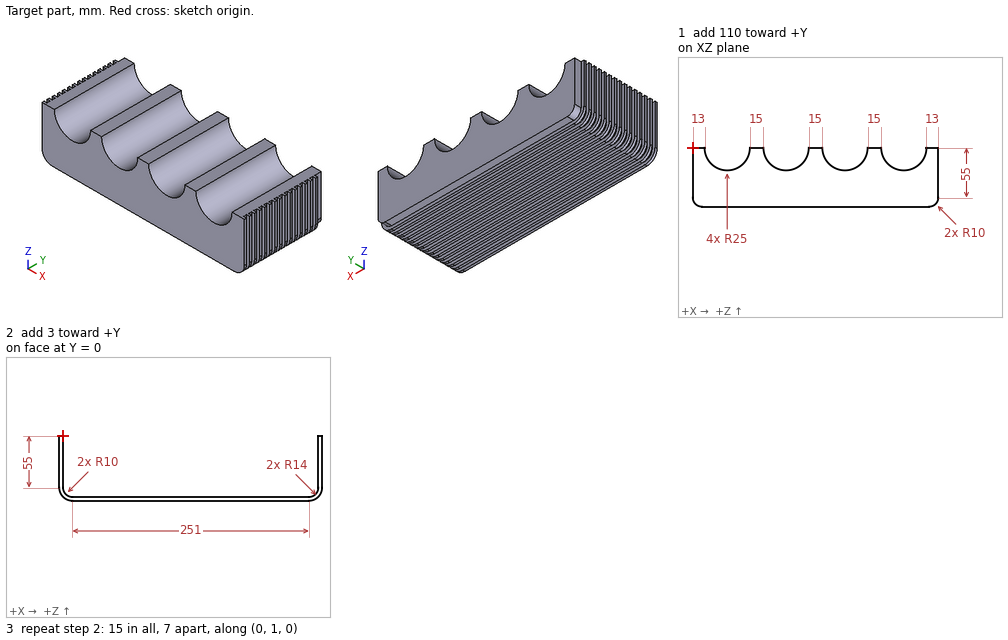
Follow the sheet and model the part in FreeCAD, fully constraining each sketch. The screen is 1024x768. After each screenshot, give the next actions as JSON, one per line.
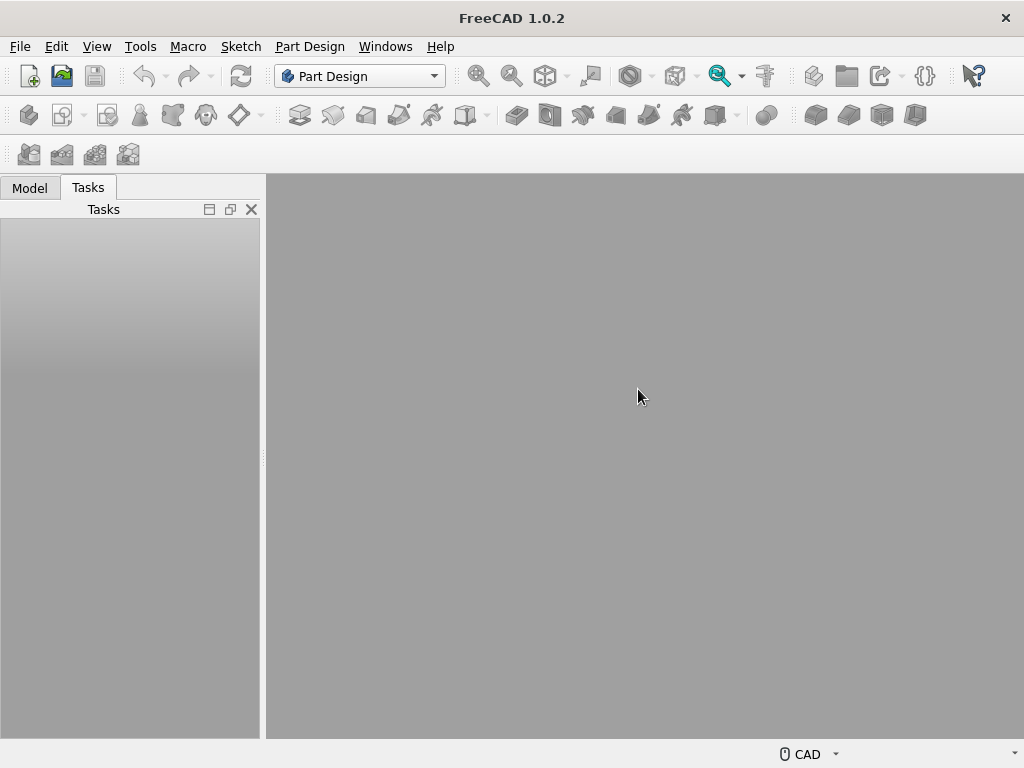
{"action": "left_click", "coordinate": [29, 76]}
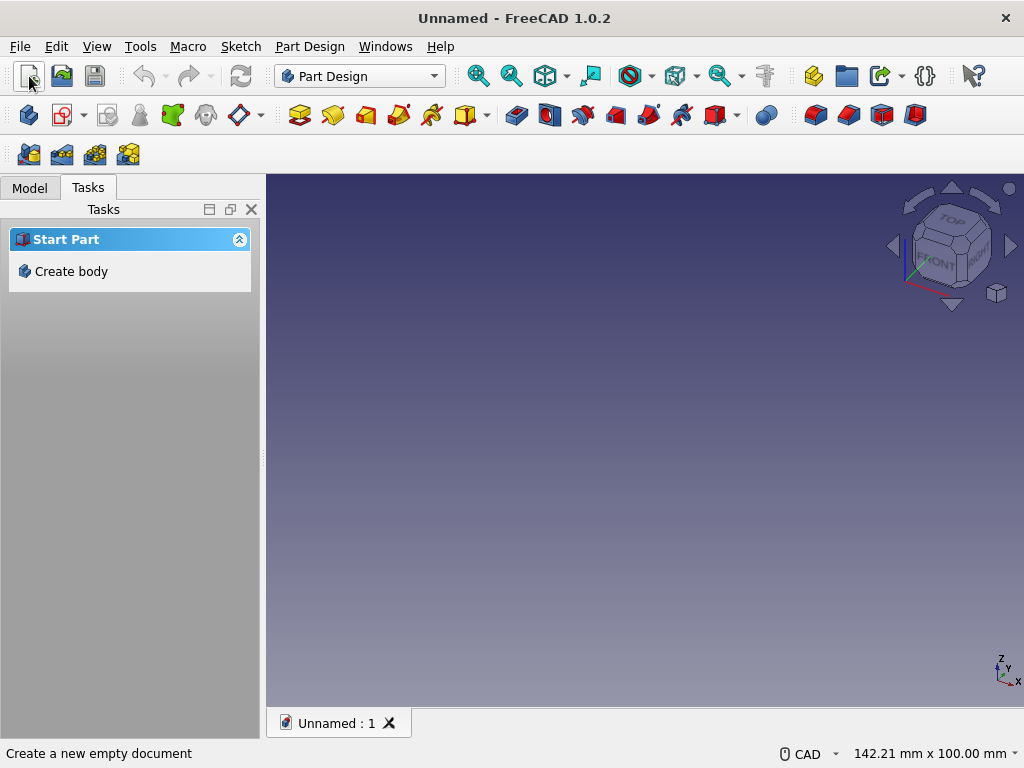
{"action": "left_click", "coordinate": [62, 116]}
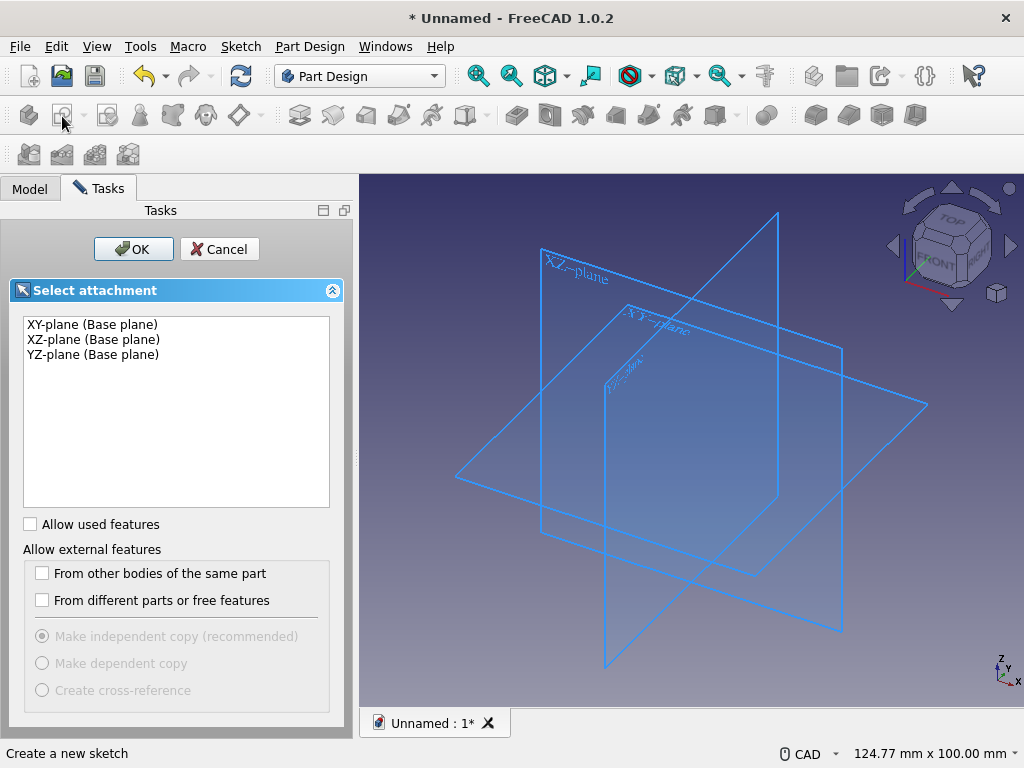
{"action": "left_click", "coordinate": [84, 340]}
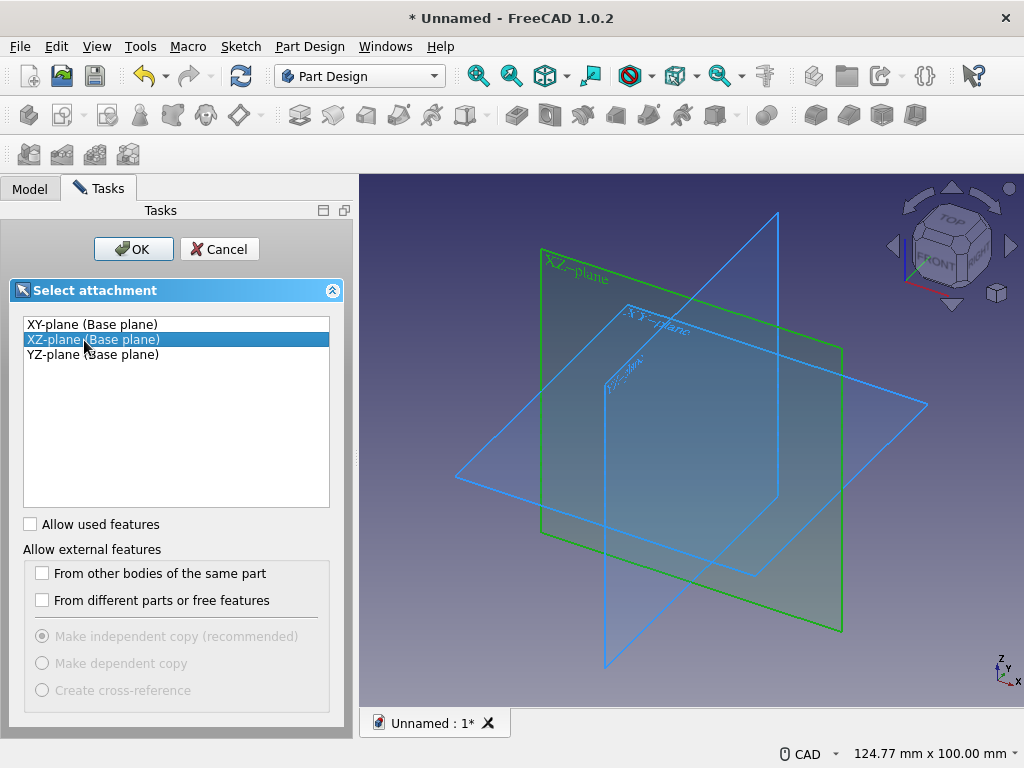
{"action": "left_click", "coordinate": [134, 249]}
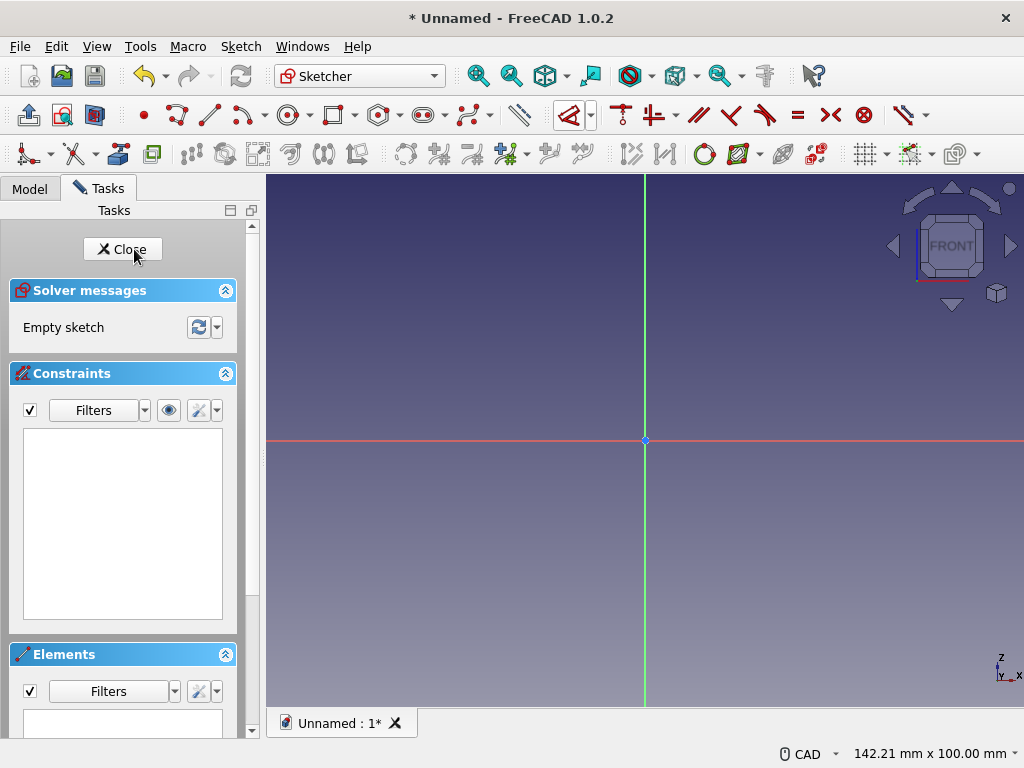
{"action": "scroll", "coordinate": [318, 384], "scroll_direction": "down", "scroll_amount": 7}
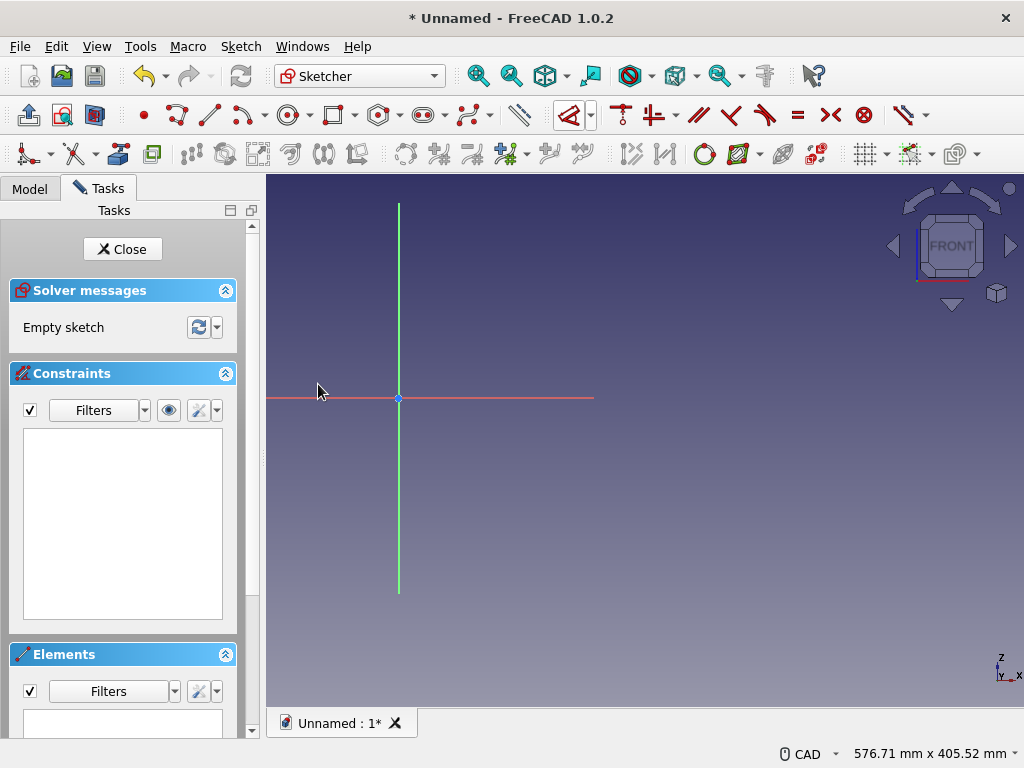
{"action": "left_click", "coordinate": [210, 116]}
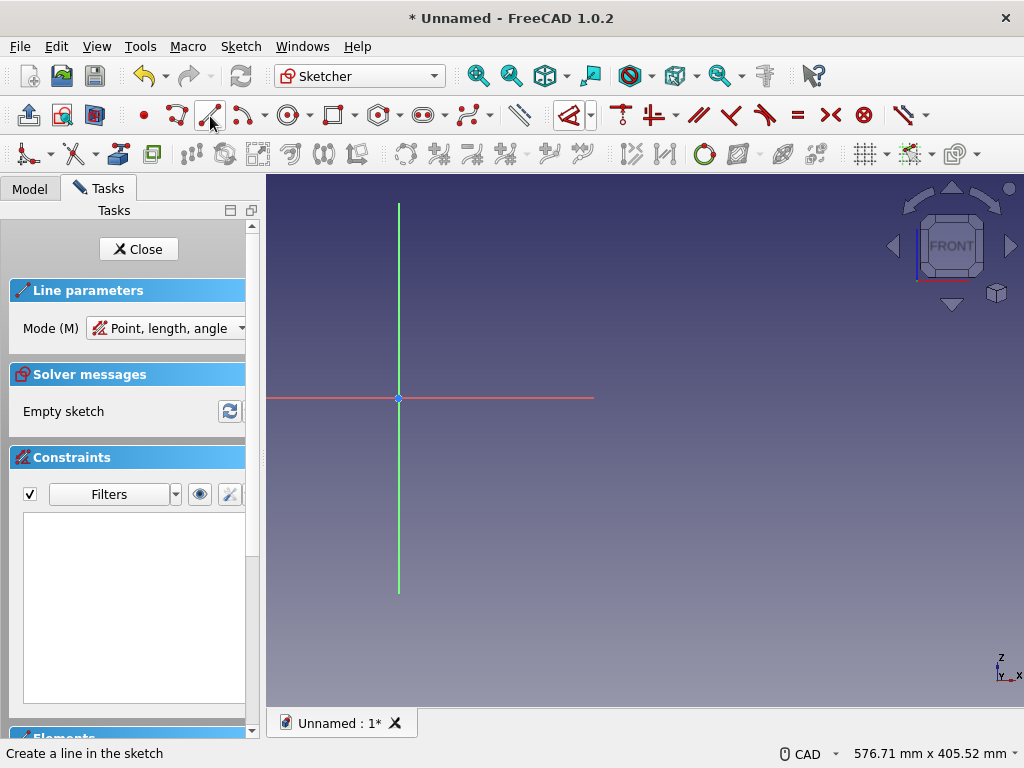
{"action": "left_click", "coordinate": [481, 398]}
{"action": "left_click", "coordinate": [501, 407]}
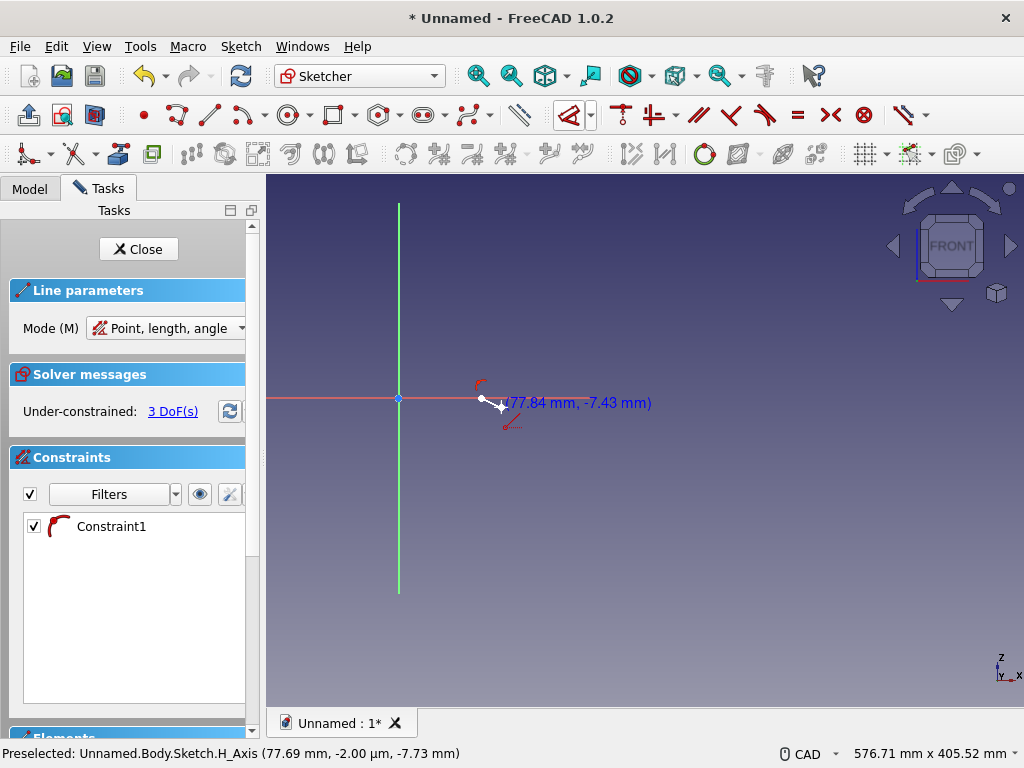
{"action": "left_click", "coordinate": [567, 398]}
{"action": "left_click", "coordinate": [587, 407]}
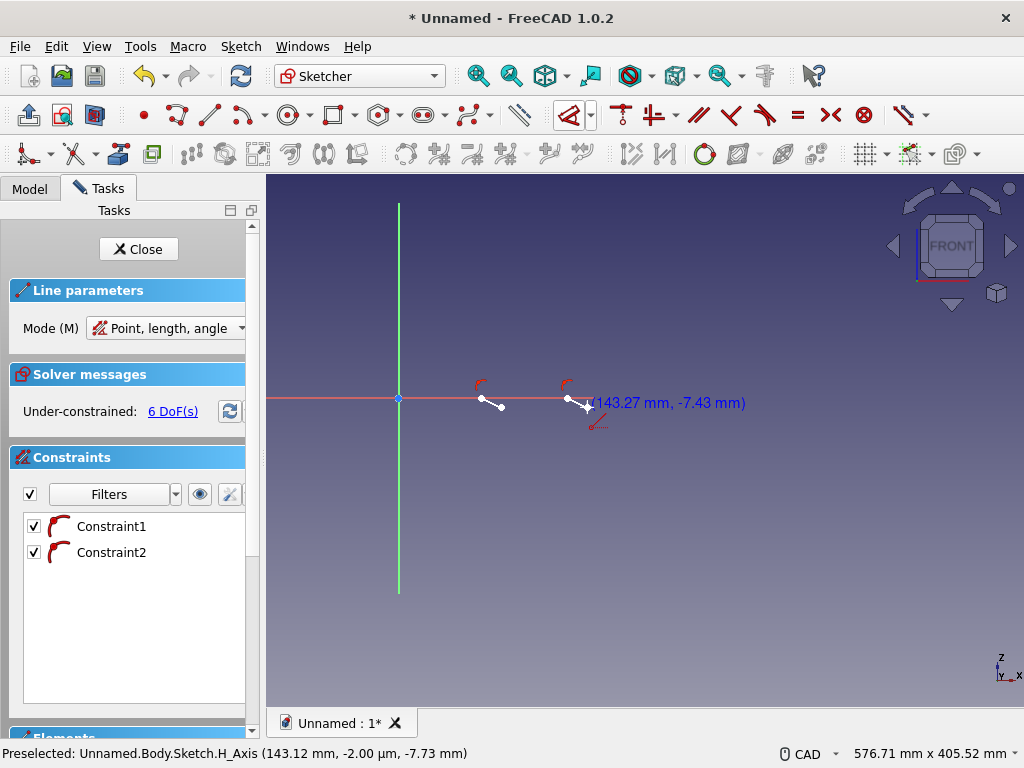
{"action": "left_click", "coordinate": [652, 398]}
{"action": "left_click", "coordinate": [672, 407]}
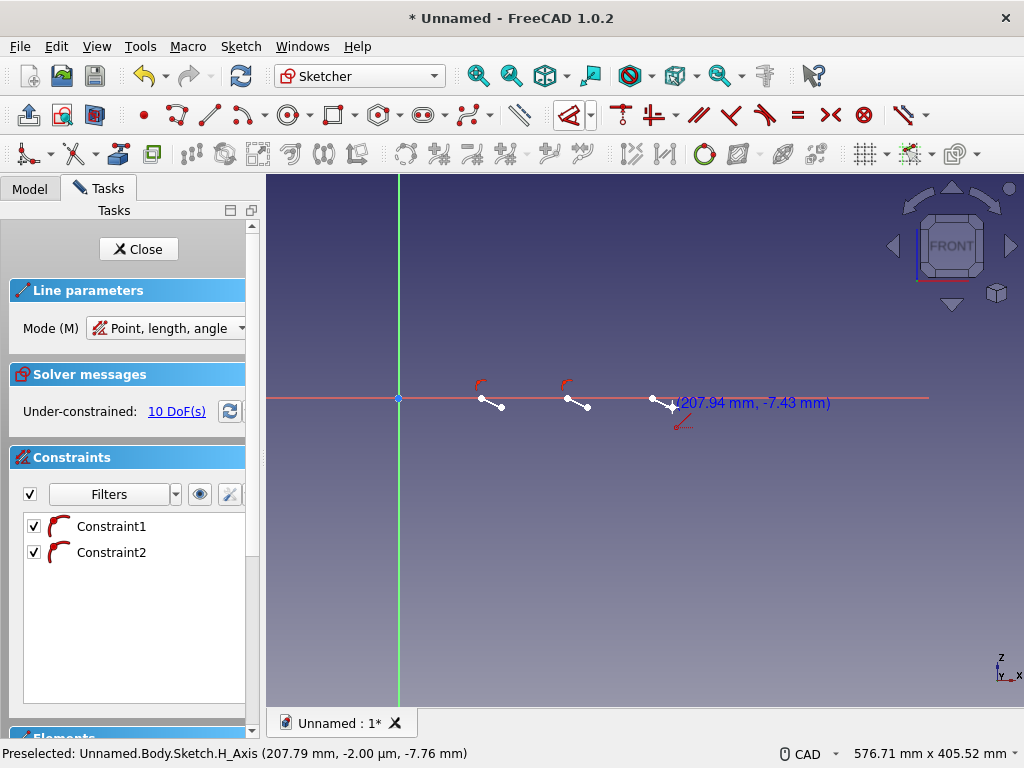
{"action": "left_click", "coordinate": [177, 116]}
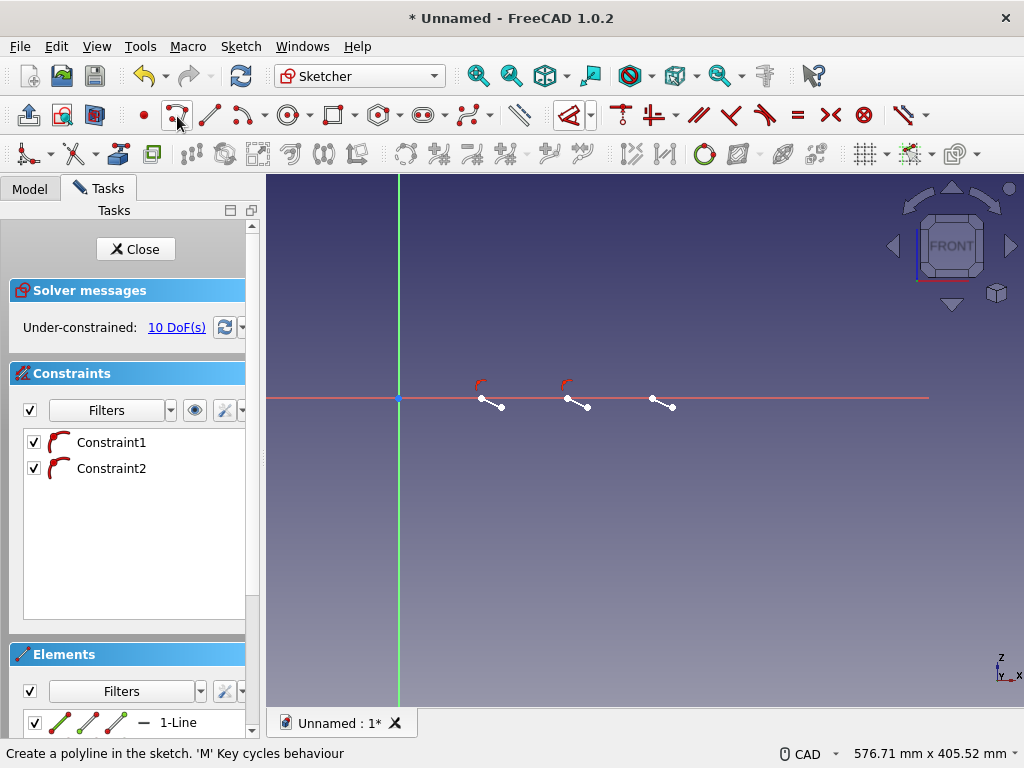
{"action": "left_click", "coordinate": [738, 398]}
{"action": "left_click", "coordinate": [755, 407]}
{"action": "left_click", "coordinate": [755, 471]}
{"action": "right_click", "coordinate": [755, 471]}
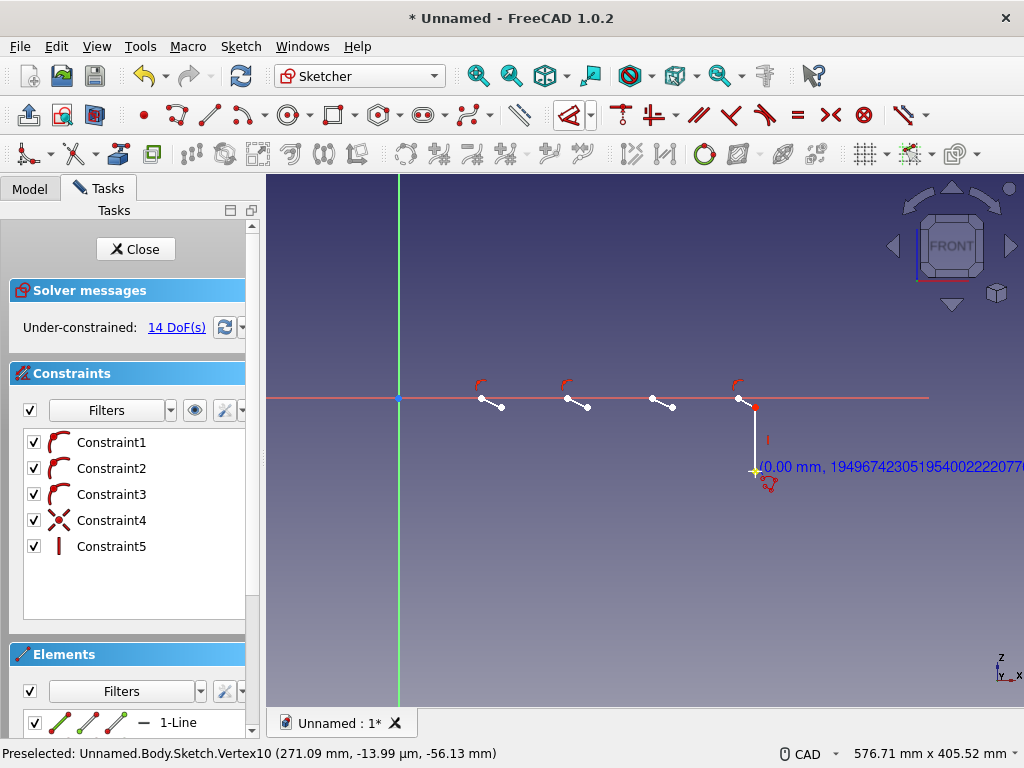
{"action": "left_click", "coordinate": [210, 116]}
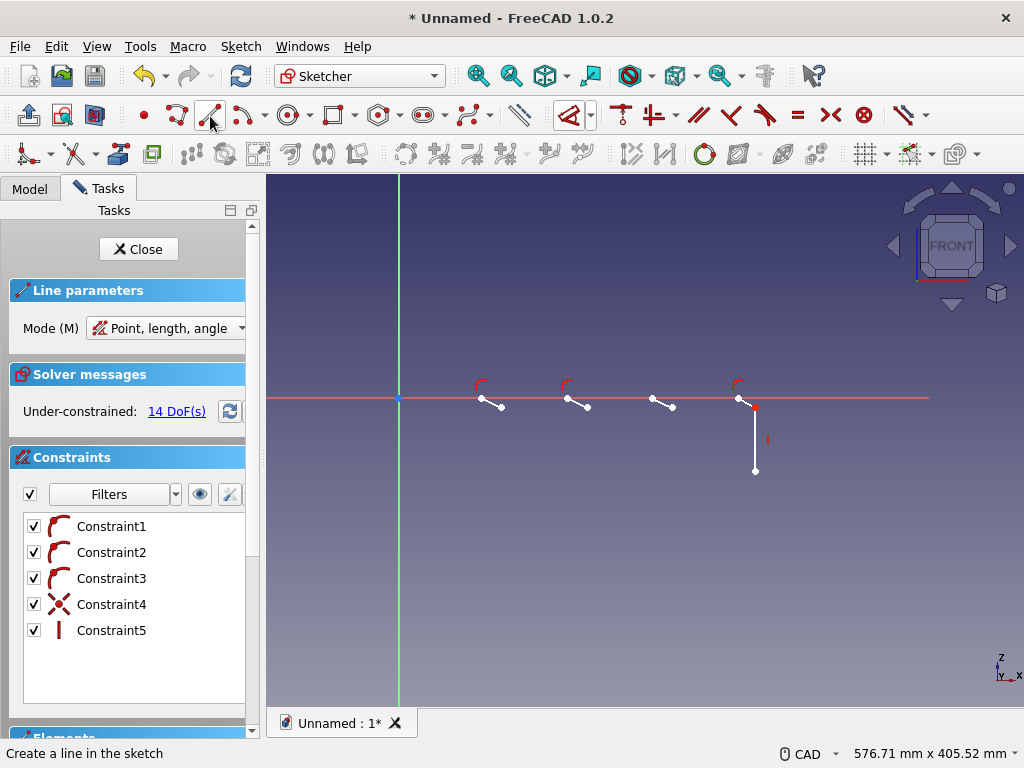
{"action": "left_click", "coordinate": [742, 484]}
{"action": "left_click", "coordinate": [412, 484]}